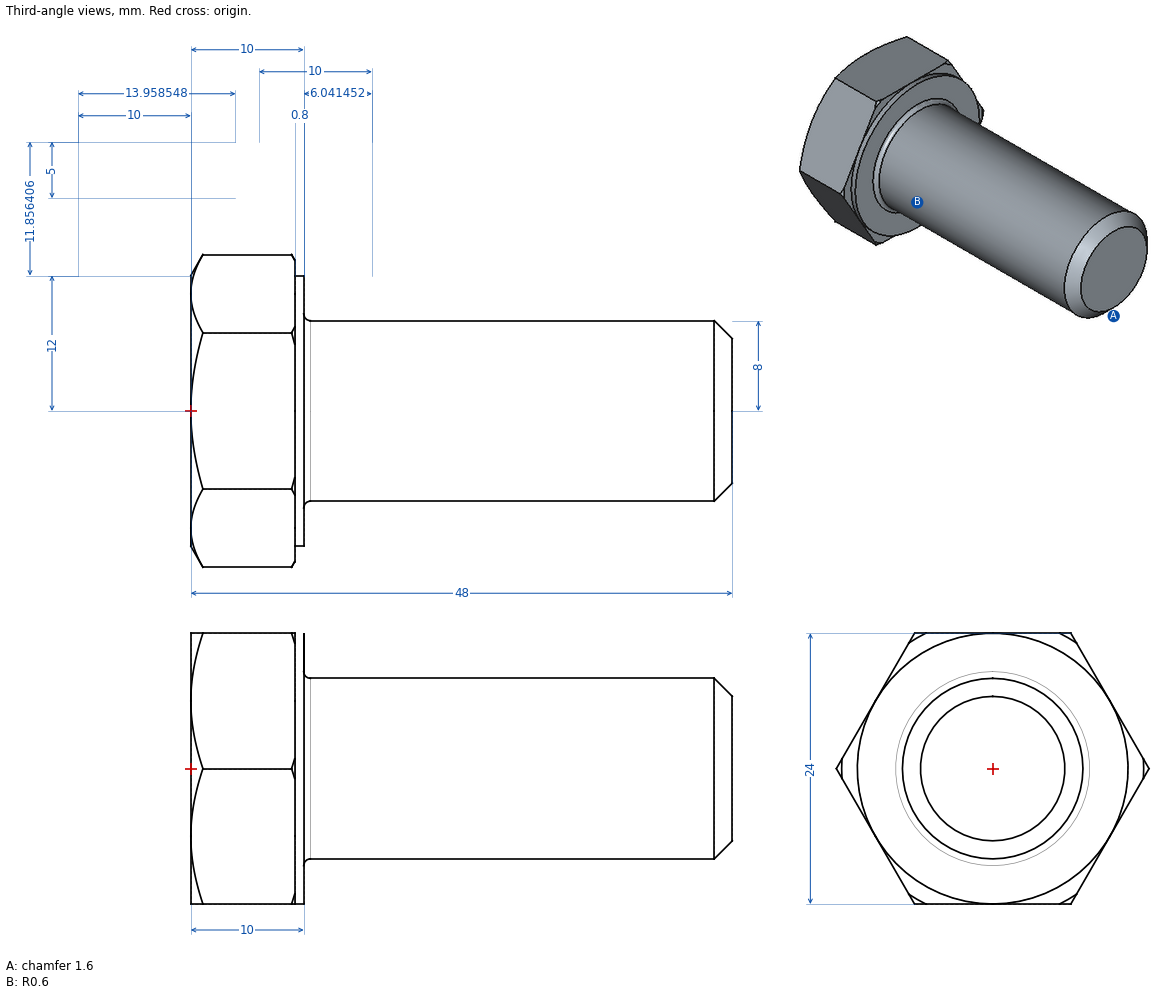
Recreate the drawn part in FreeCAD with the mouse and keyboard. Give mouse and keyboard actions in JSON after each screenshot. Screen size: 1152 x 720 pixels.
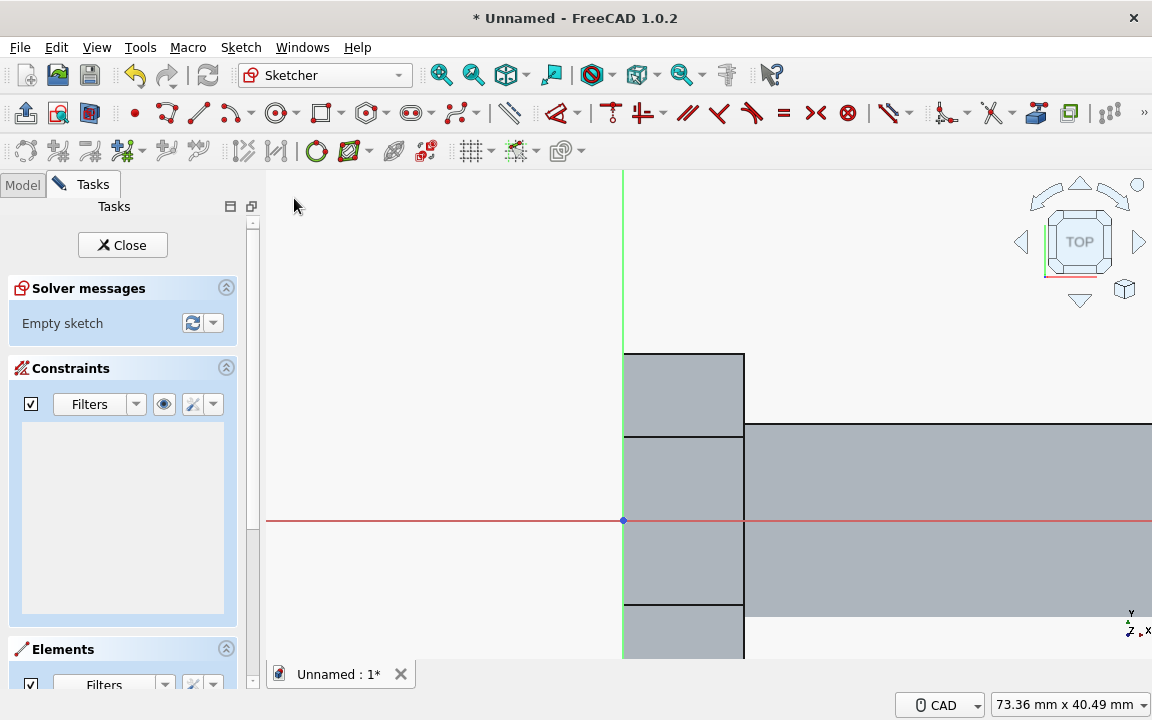
{"action": "left_click", "coordinate": [168, 114]}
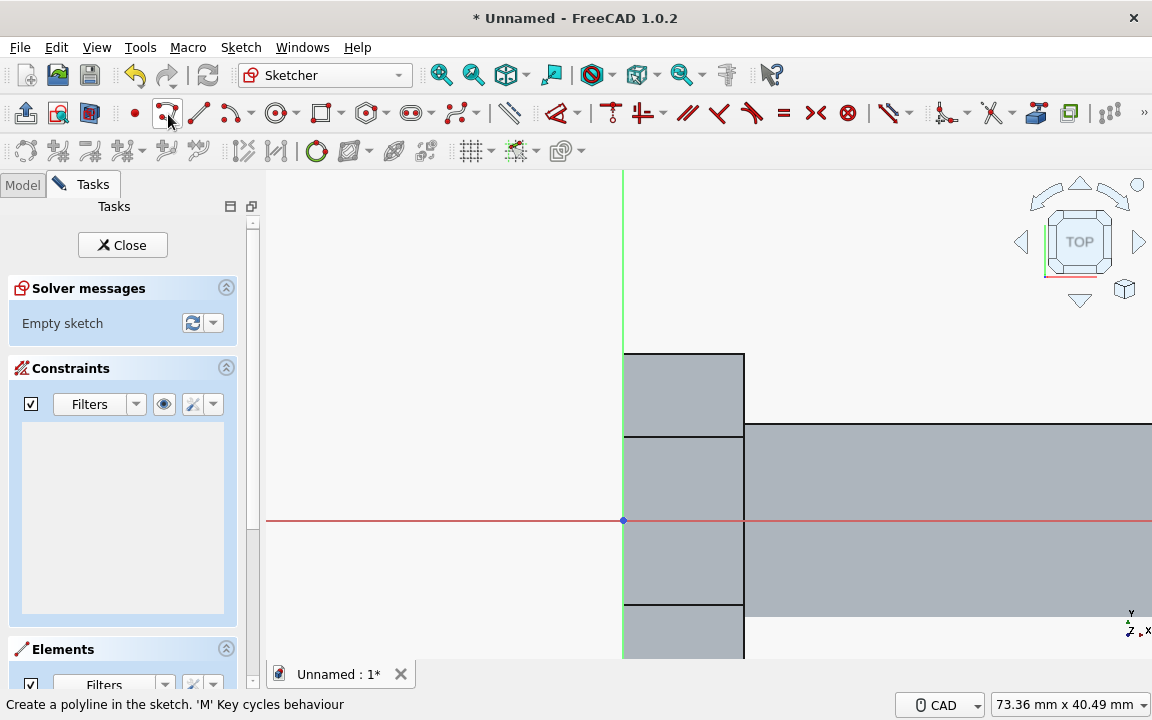
{"action": "left_click", "coordinate": [623, 376]}
{"action": "left_click", "coordinate": [671, 293]}
{"action": "left_click", "coordinate": [671, 233]}
{"action": "left_click", "coordinate": [502, 233]}
{"action": "left_click", "coordinate": [502, 376]}
{"action": "left_click", "coordinate": [623, 377]}
{"action": "key", "text": "Escape"}
{"action": "key", "text": "Escape"}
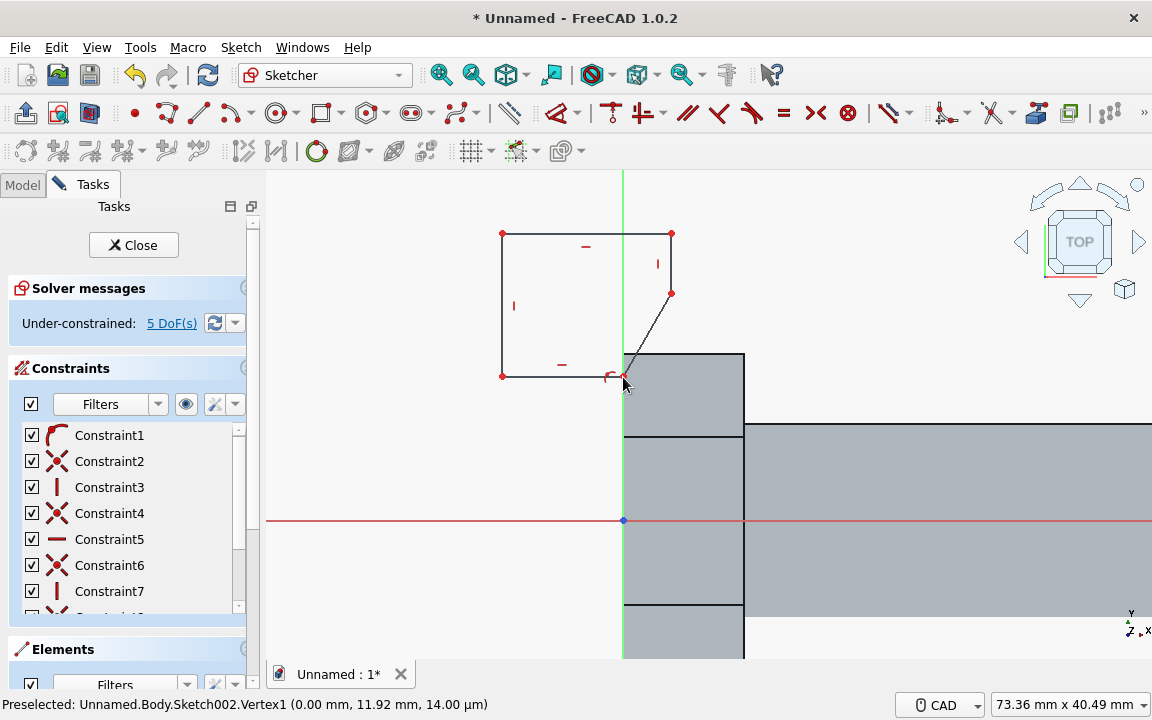
{"action": "left_click", "coordinate": [556, 114]}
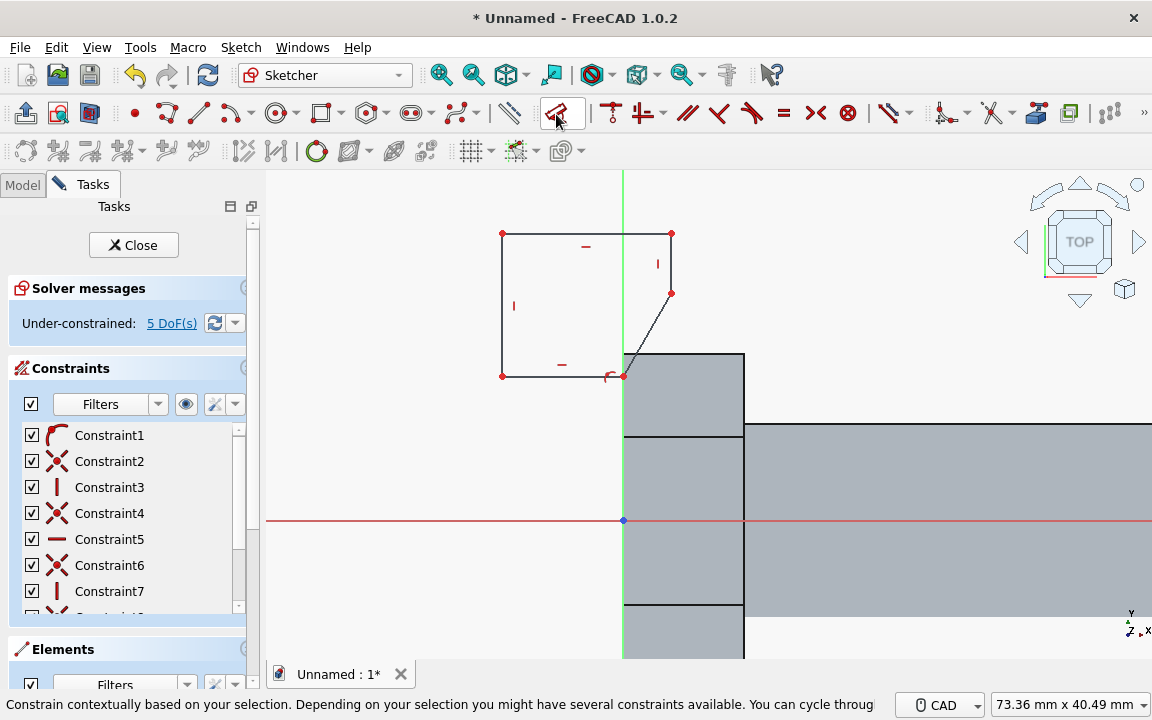
{"action": "left_click", "coordinate": [671, 276]}
{"action": "left_click", "coordinate": [705, 264]}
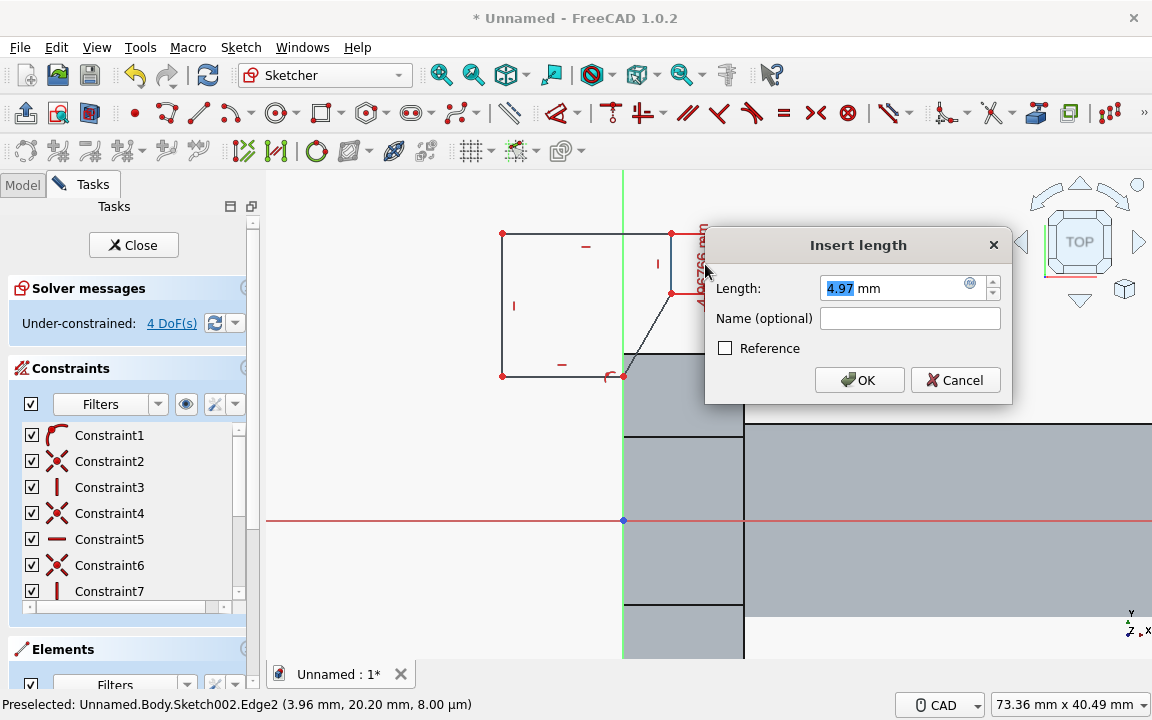
{"action": "type", "text": "5"}
{"action": "key", "text": "Return"}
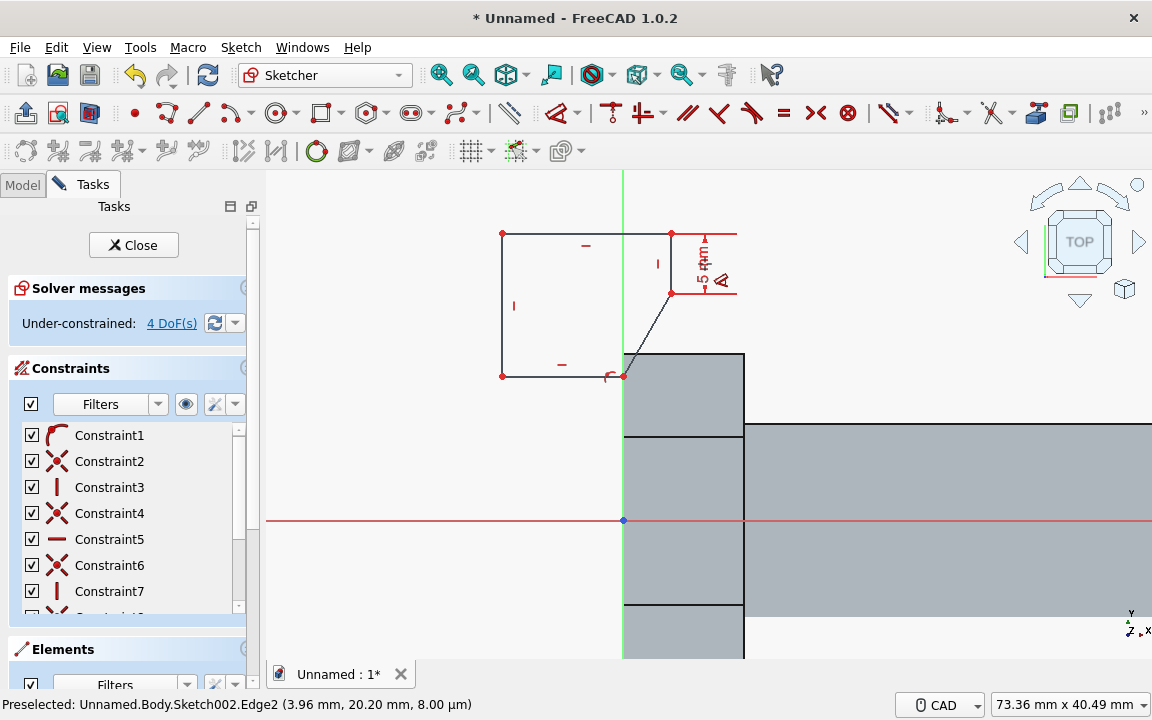
{"action": "left_click", "coordinate": [538, 377]}
{"action": "left_click", "coordinate": [563, 411]}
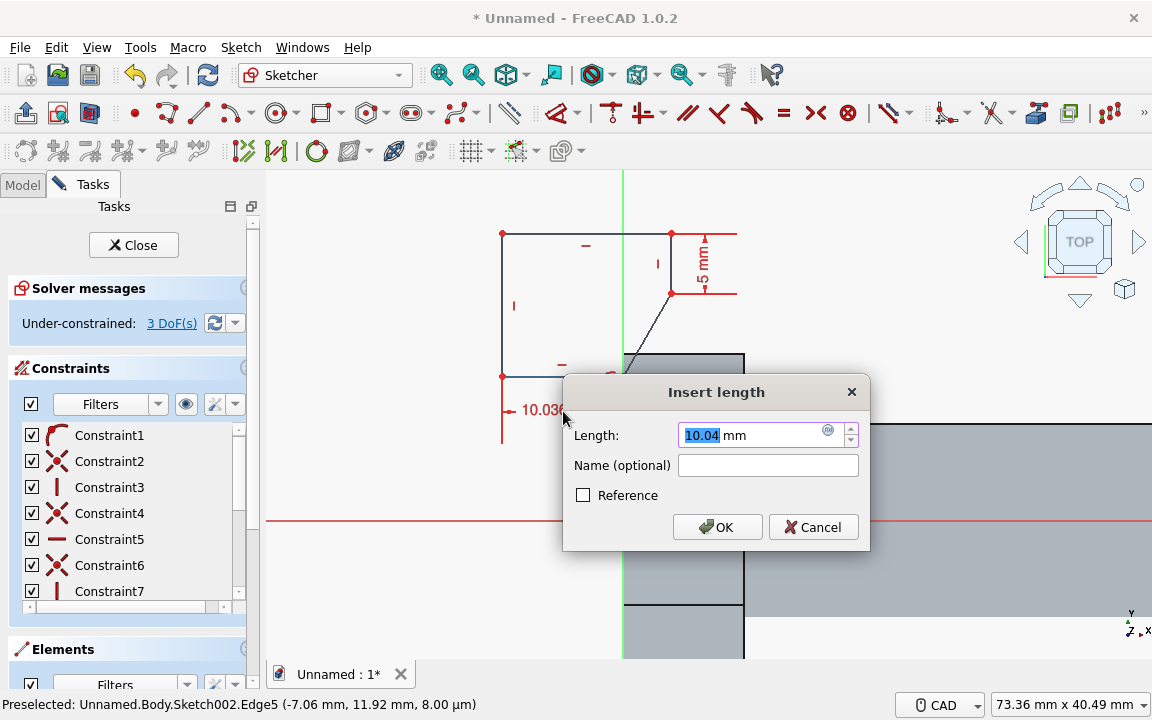
{"action": "type", "text": "10"}
{"action": "key", "text": "Return"}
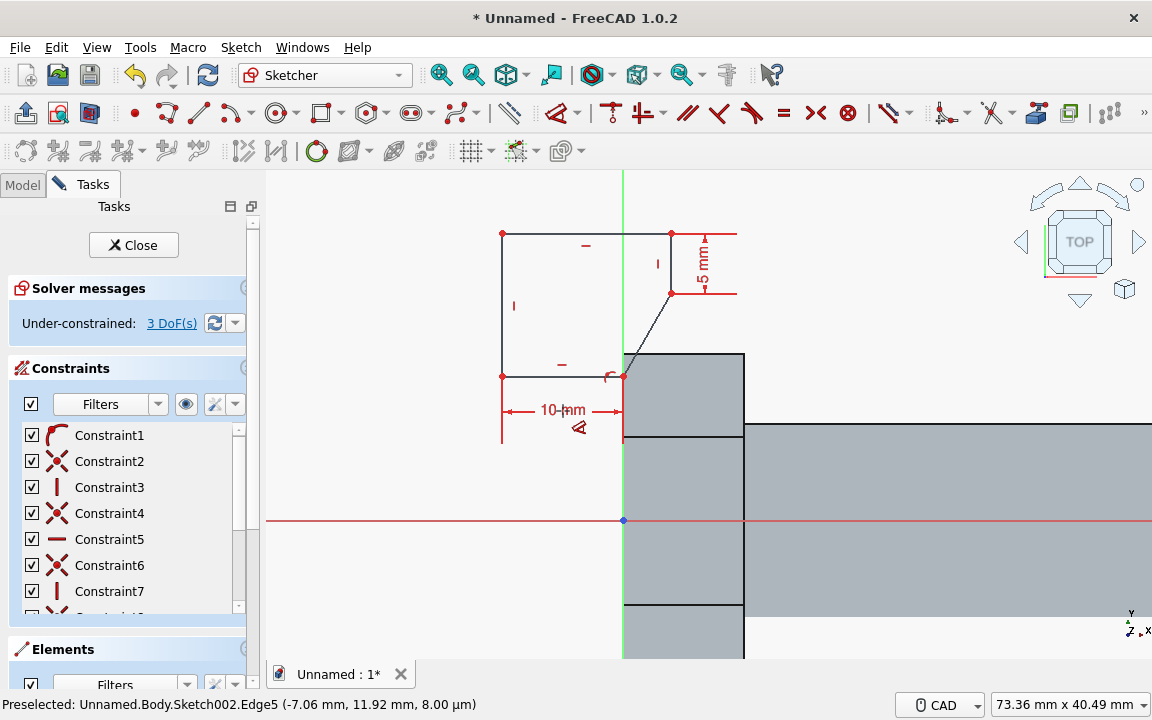
{"action": "left_click", "coordinate": [623, 377]}
{"action": "left_click", "coordinate": [657, 449]}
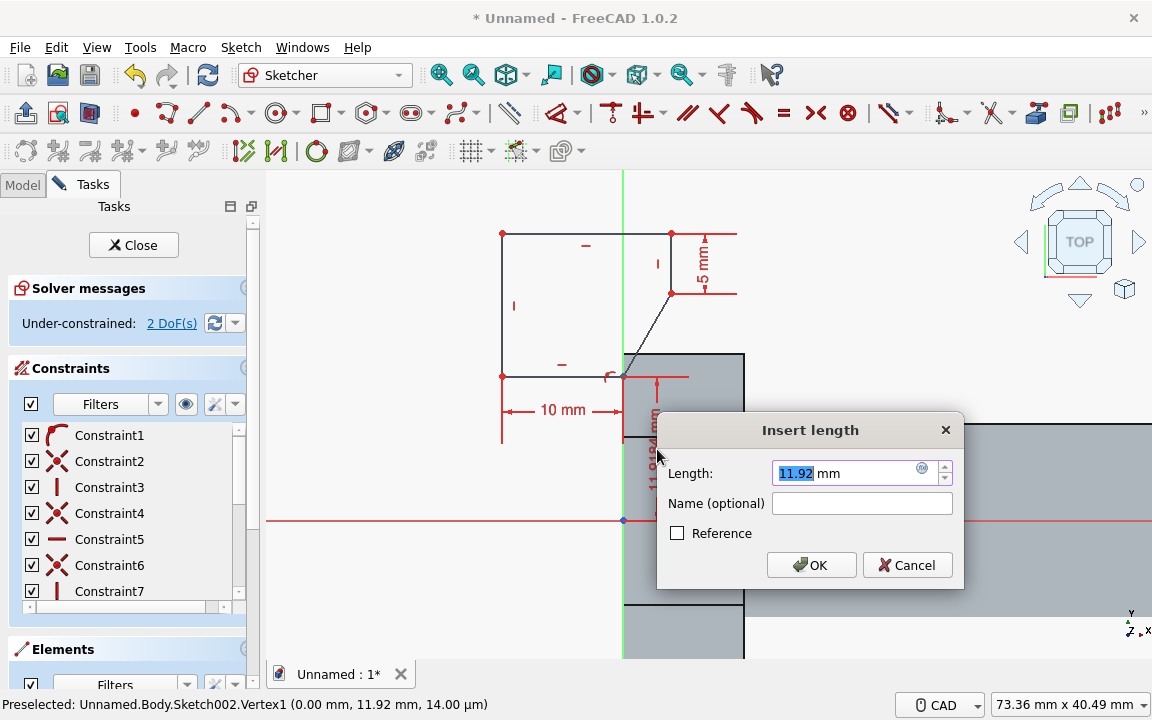
{"action": "type", "text": "12"}
{"action": "key", "text": "Return"}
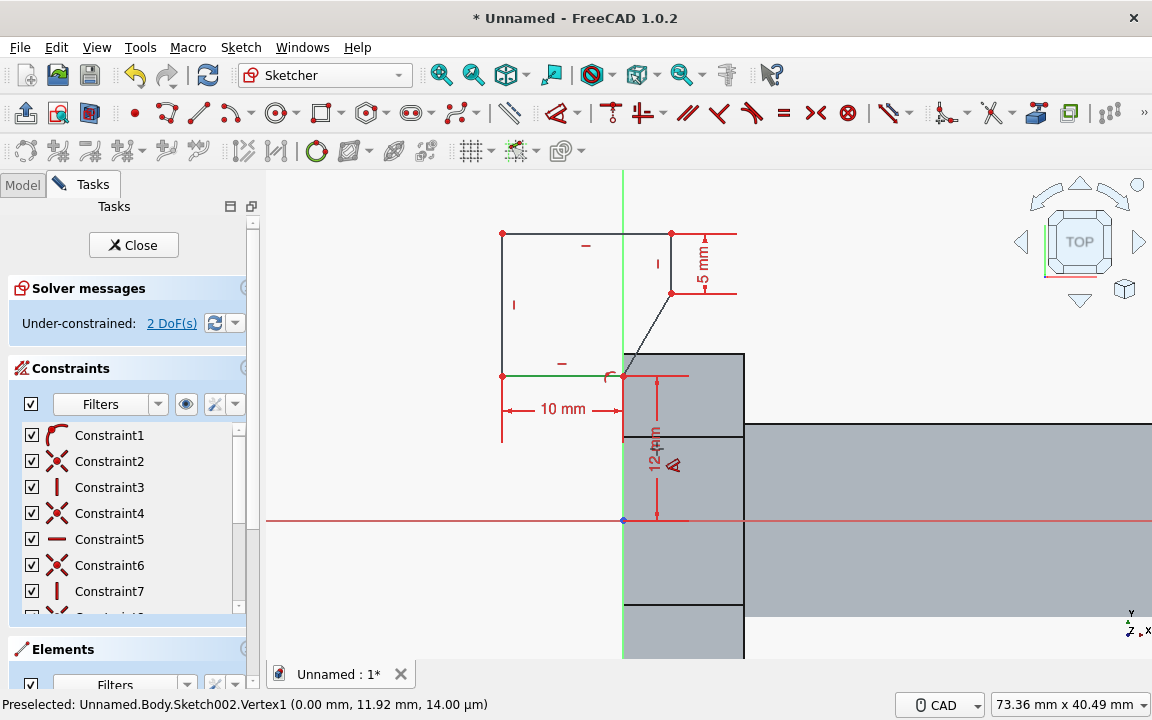
{"action": "left_click", "coordinate": [620, 234]}
{"action": "left_click", "coordinate": [587, 200]}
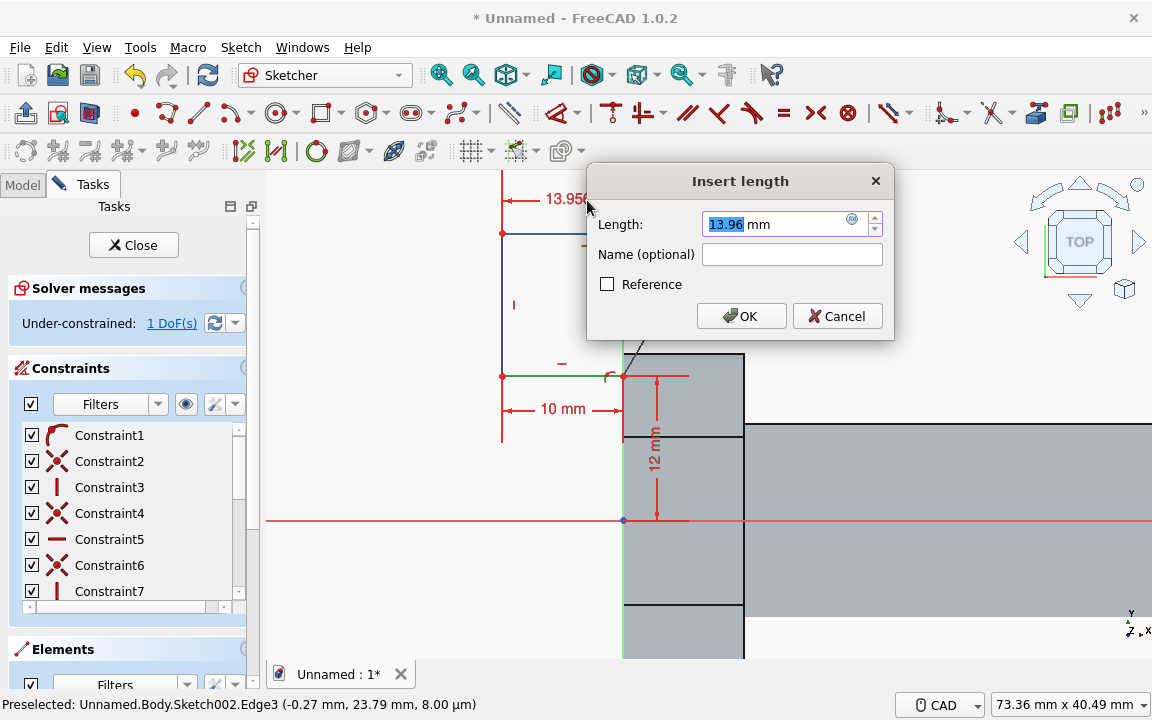
{"action": "type", "text": "13.958548"}
{"action": "key", "text": "Return"}